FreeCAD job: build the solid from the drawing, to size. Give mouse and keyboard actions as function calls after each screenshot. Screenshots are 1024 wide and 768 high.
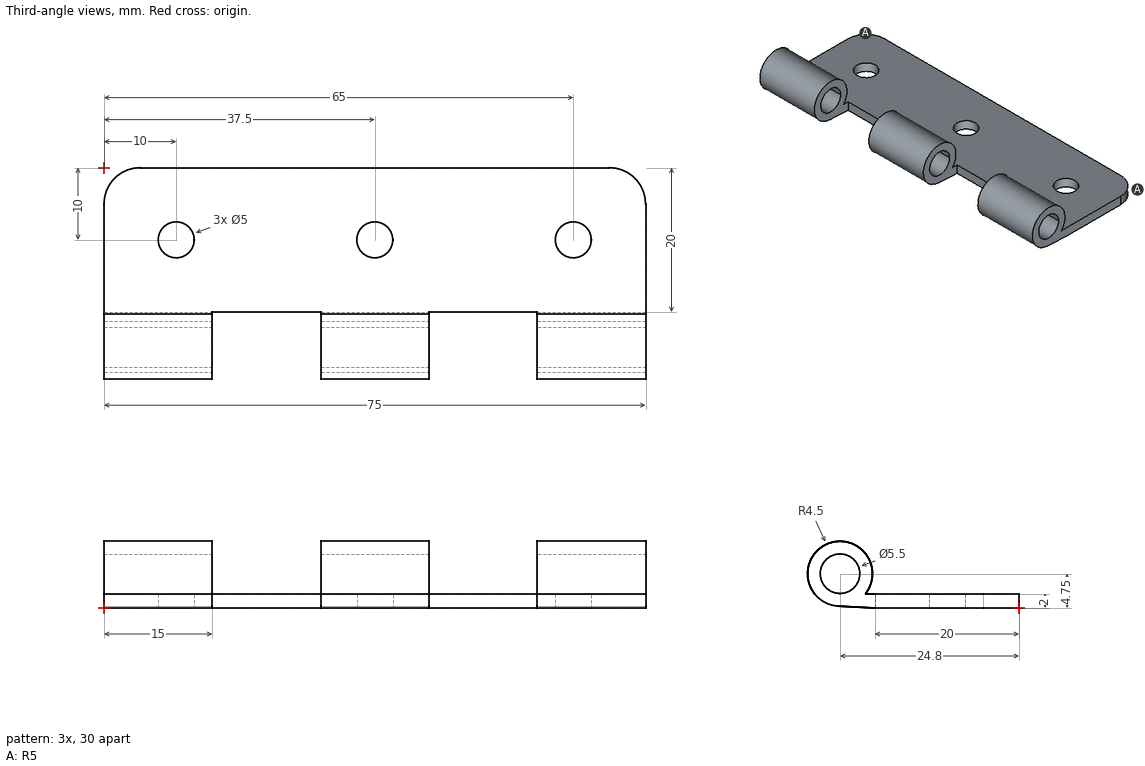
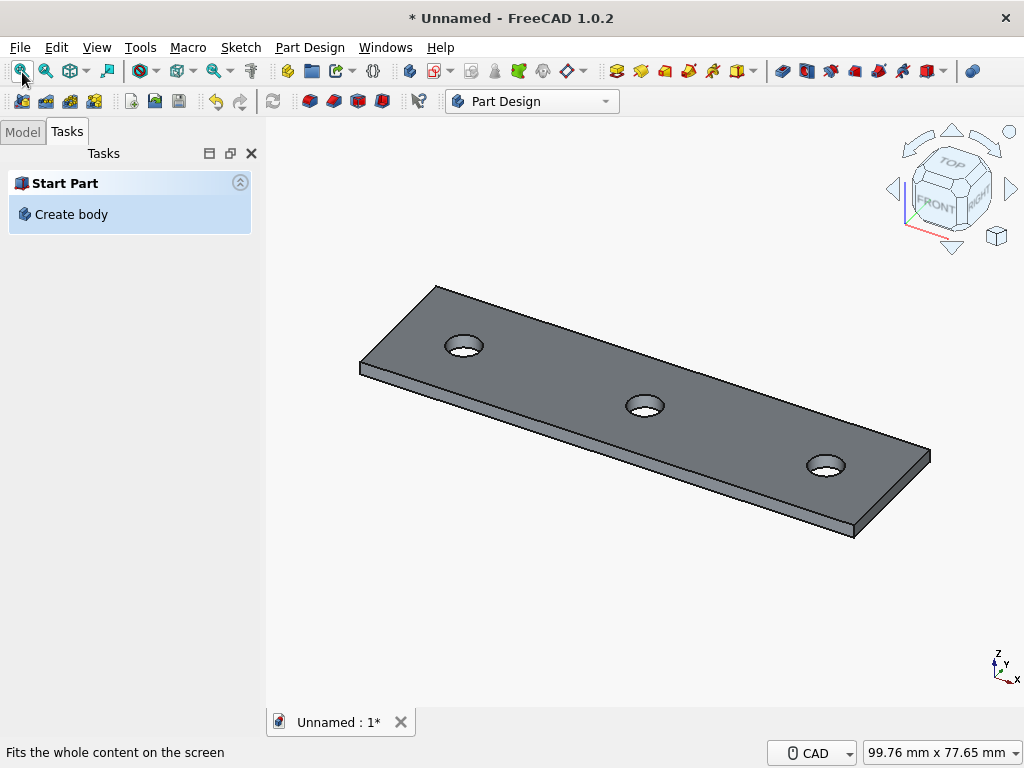
key(6)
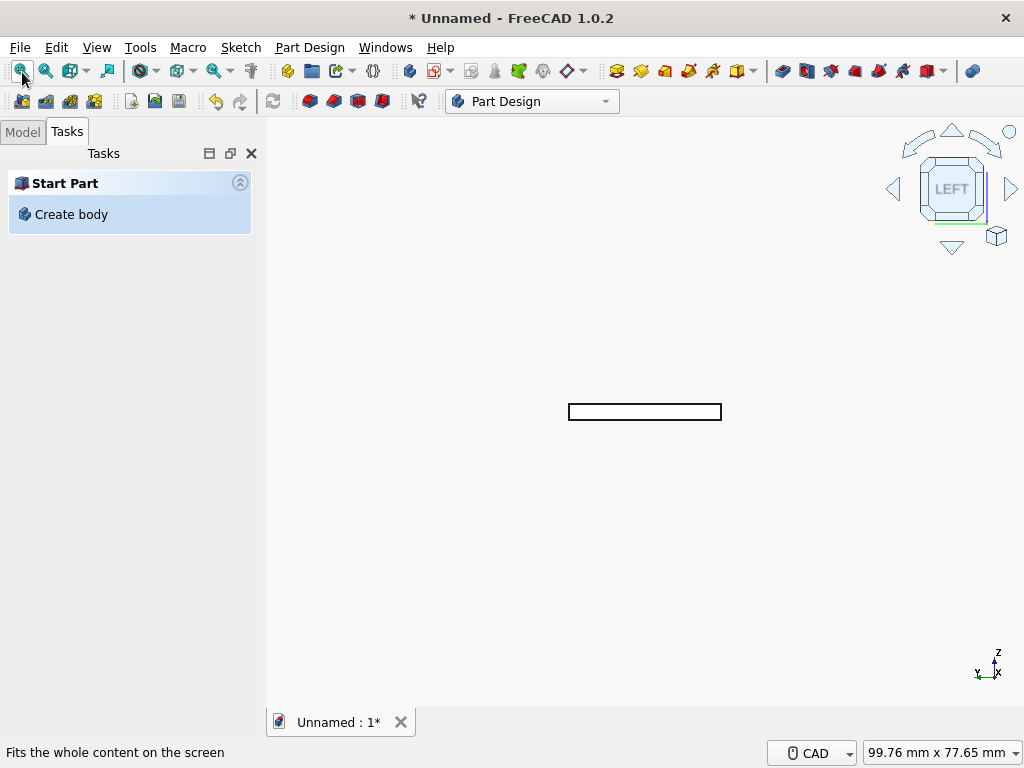
click(22, 72)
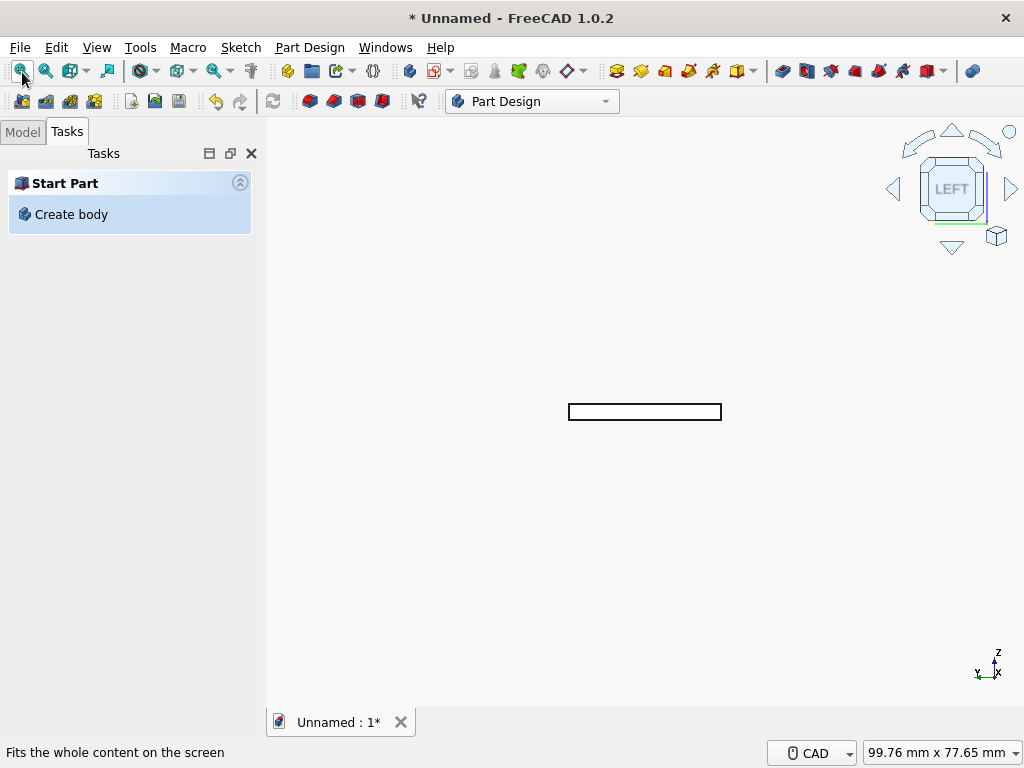
key(2)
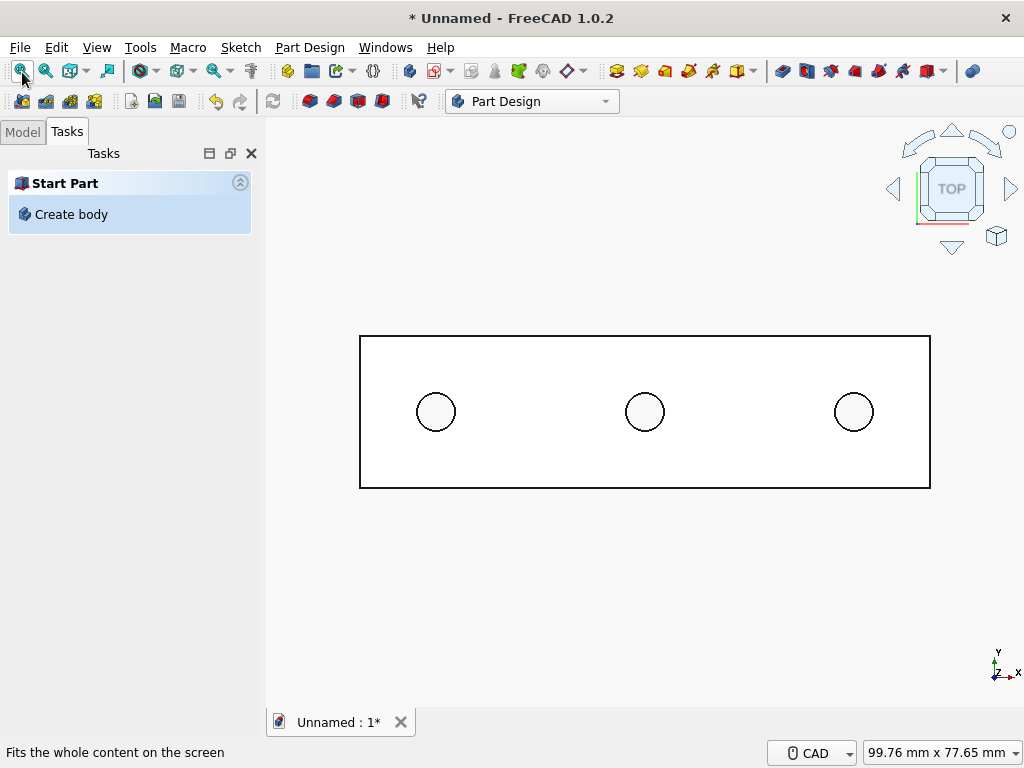
key(1)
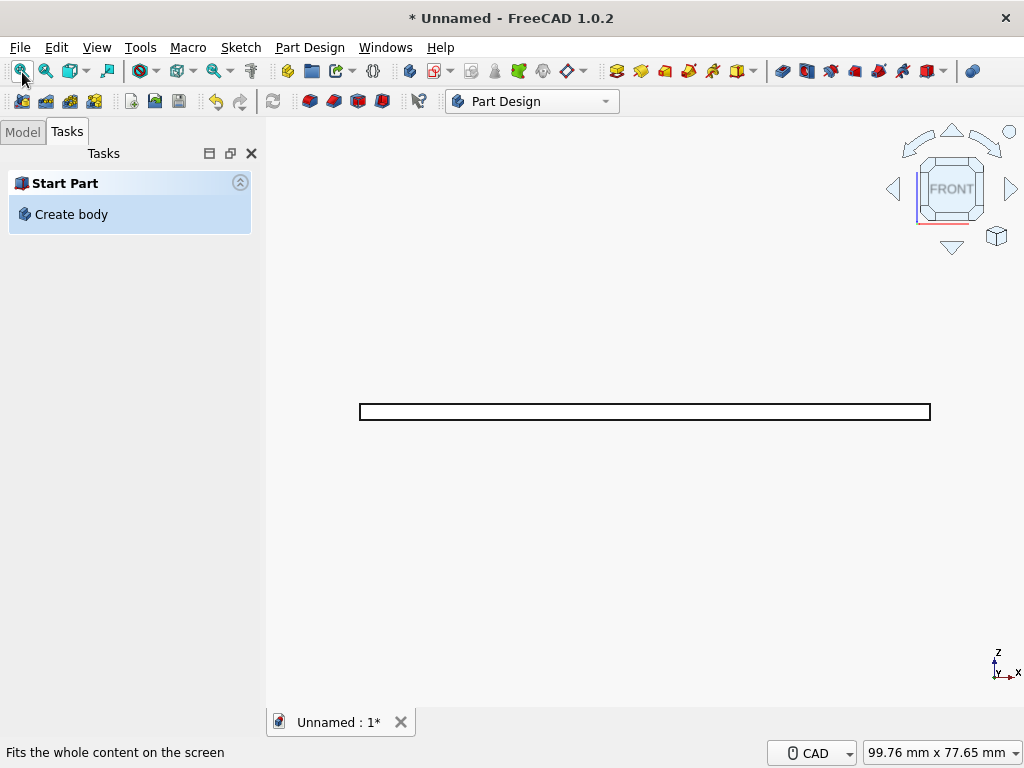
click(434, 72)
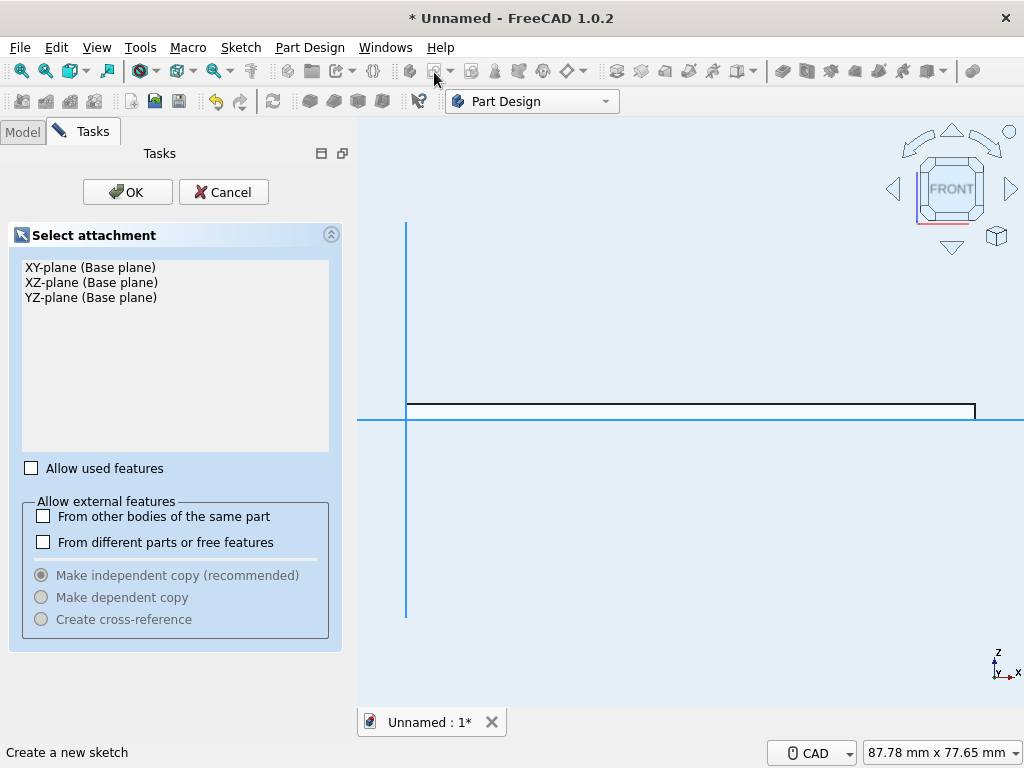
click(82, 298)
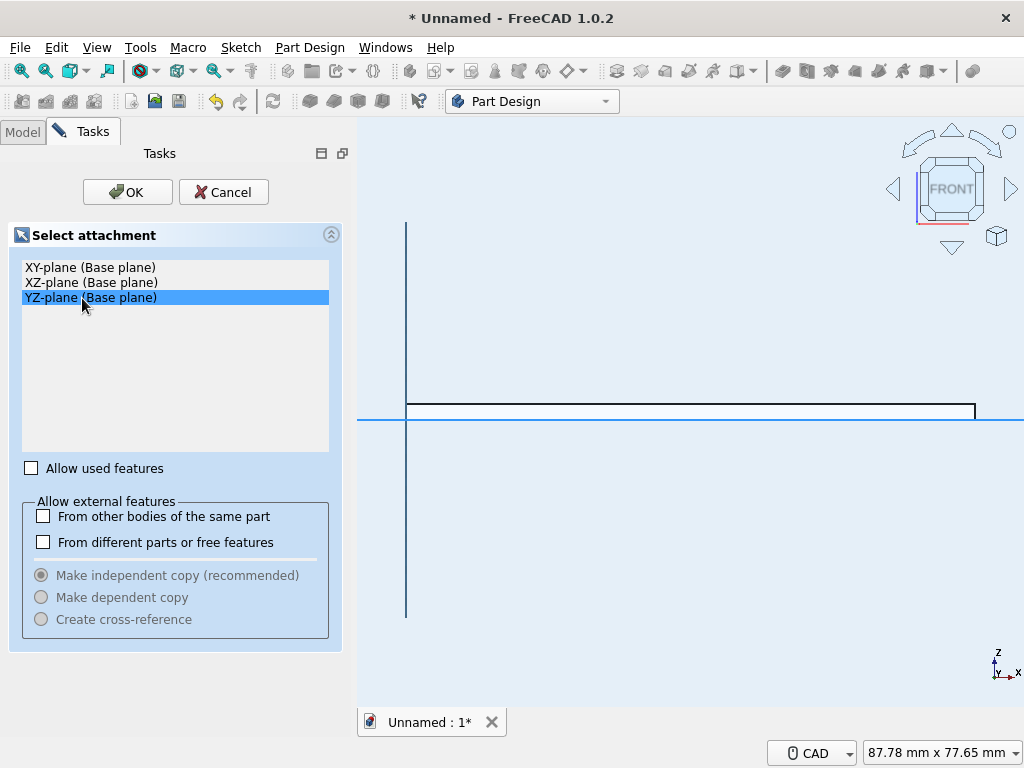
click(128, 192)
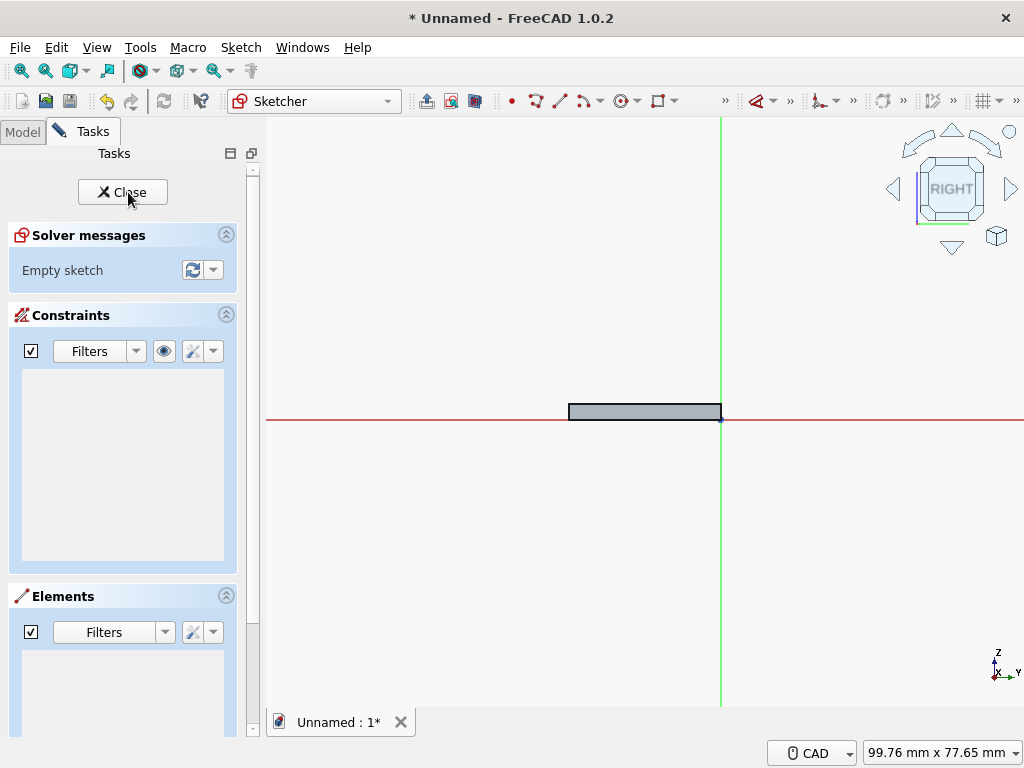
click(476, 102)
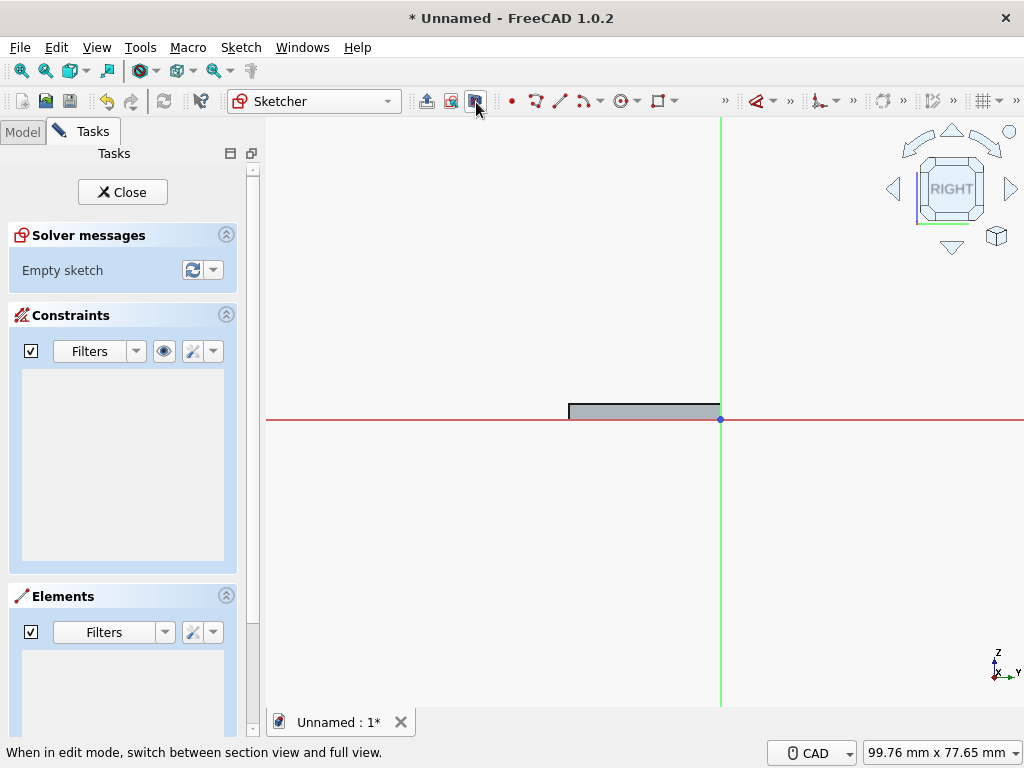
scroll(533, 381, up, 9)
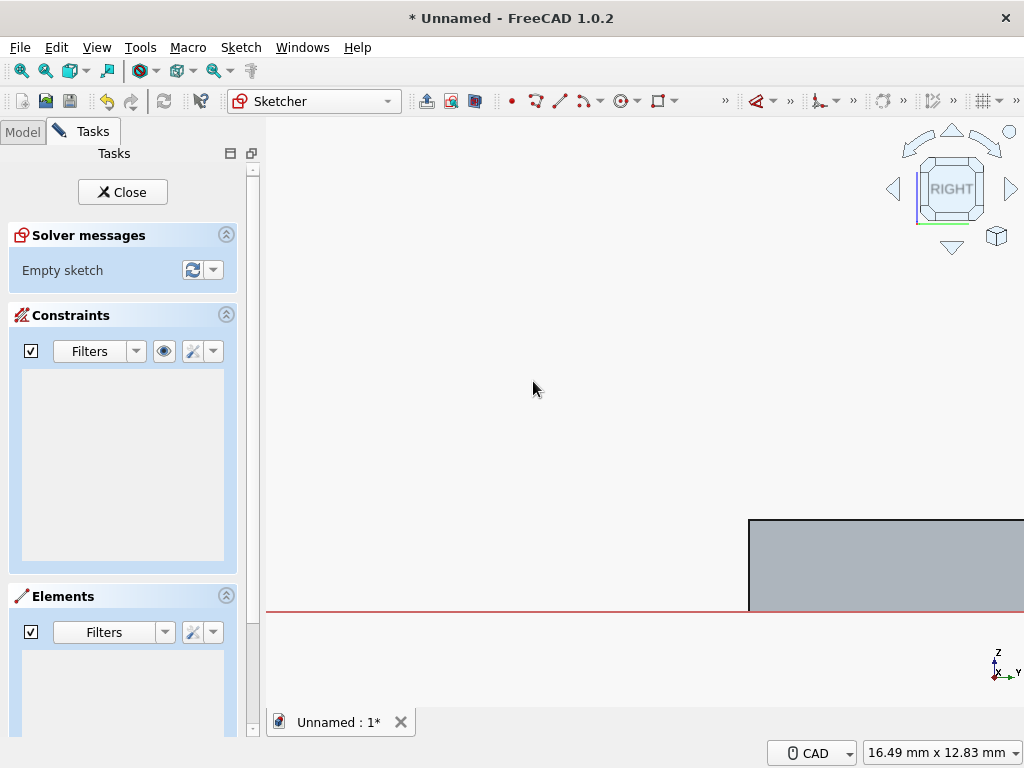
click(536, 102)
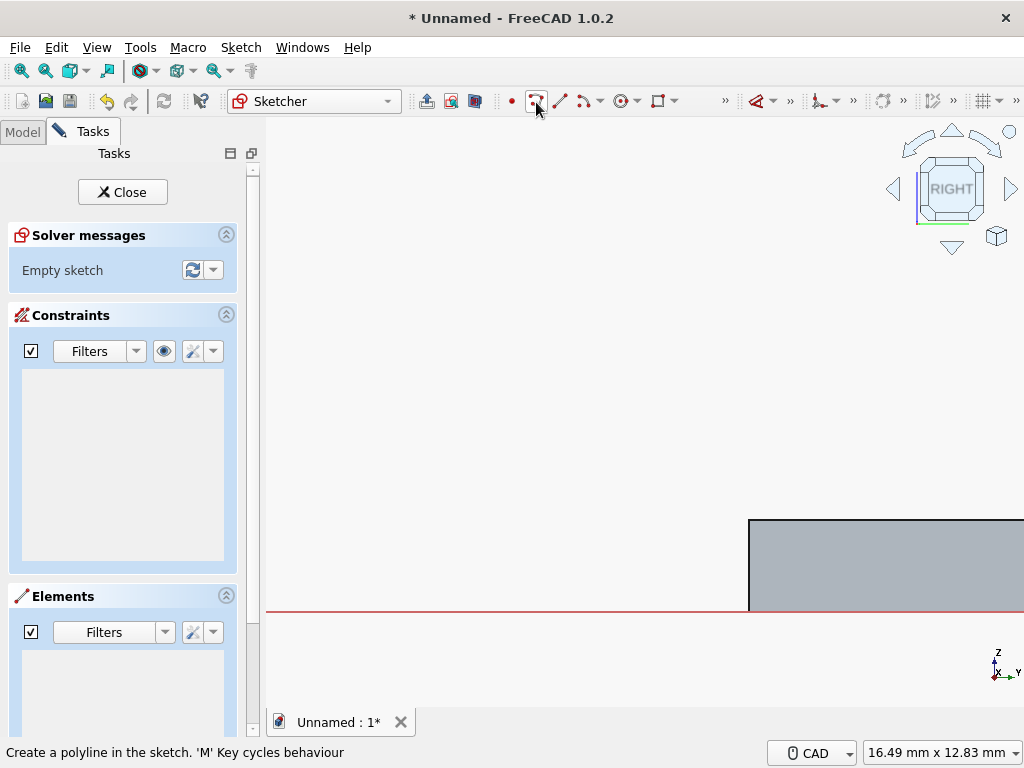
click(692, 520)
click(749, 520)
click(749, 612)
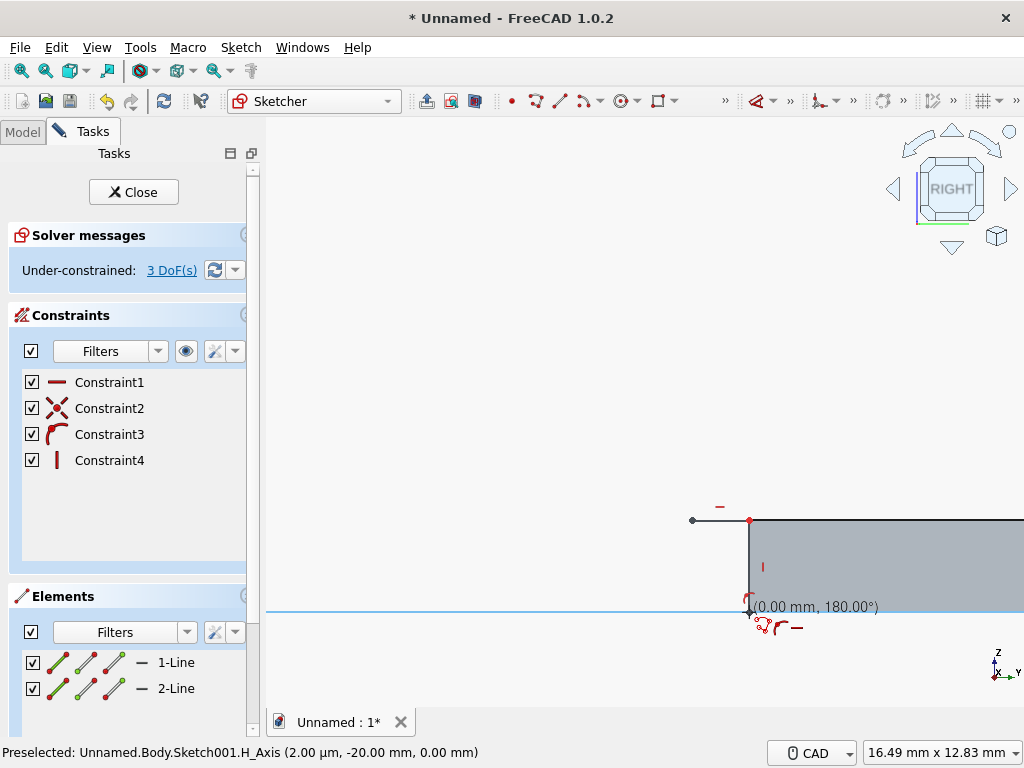
scroll(518, 600, up, 2)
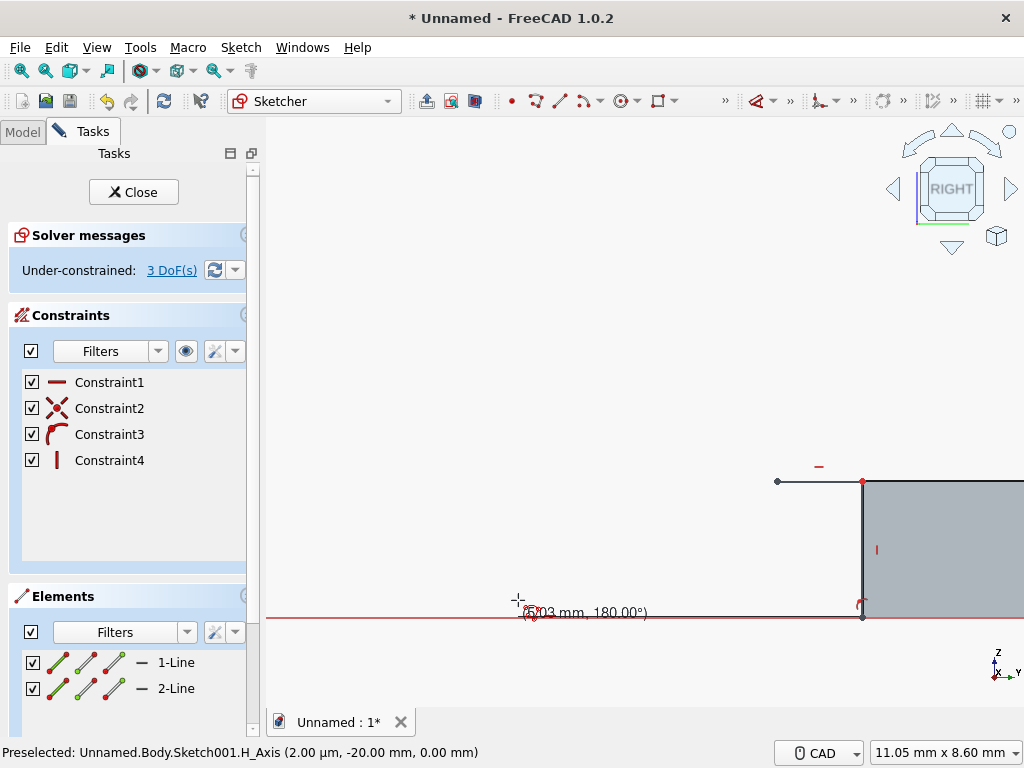
click(518, 600)
right_click(518, 600)